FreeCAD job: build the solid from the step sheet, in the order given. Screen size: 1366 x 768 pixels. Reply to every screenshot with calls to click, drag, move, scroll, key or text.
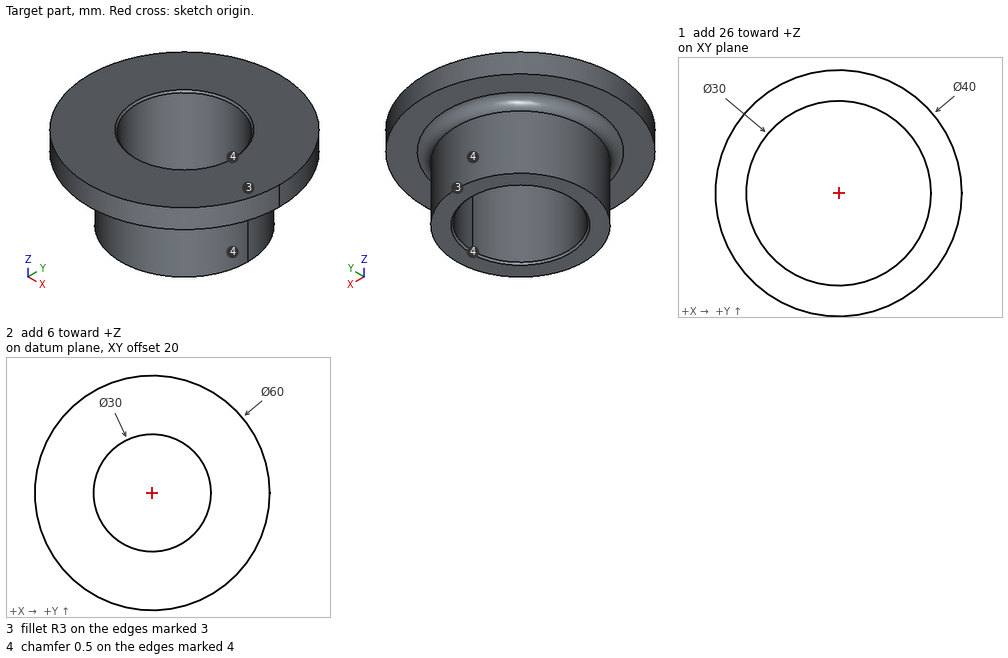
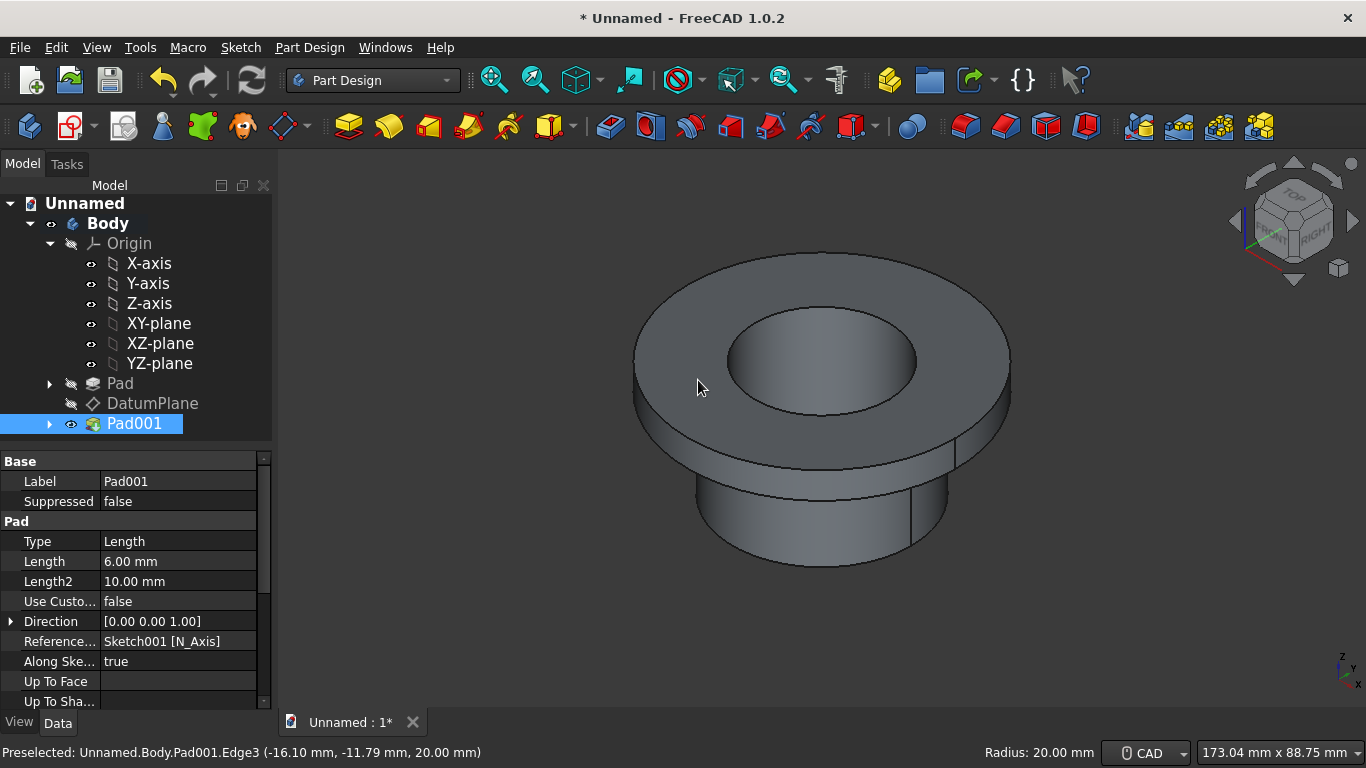
click(966, 126)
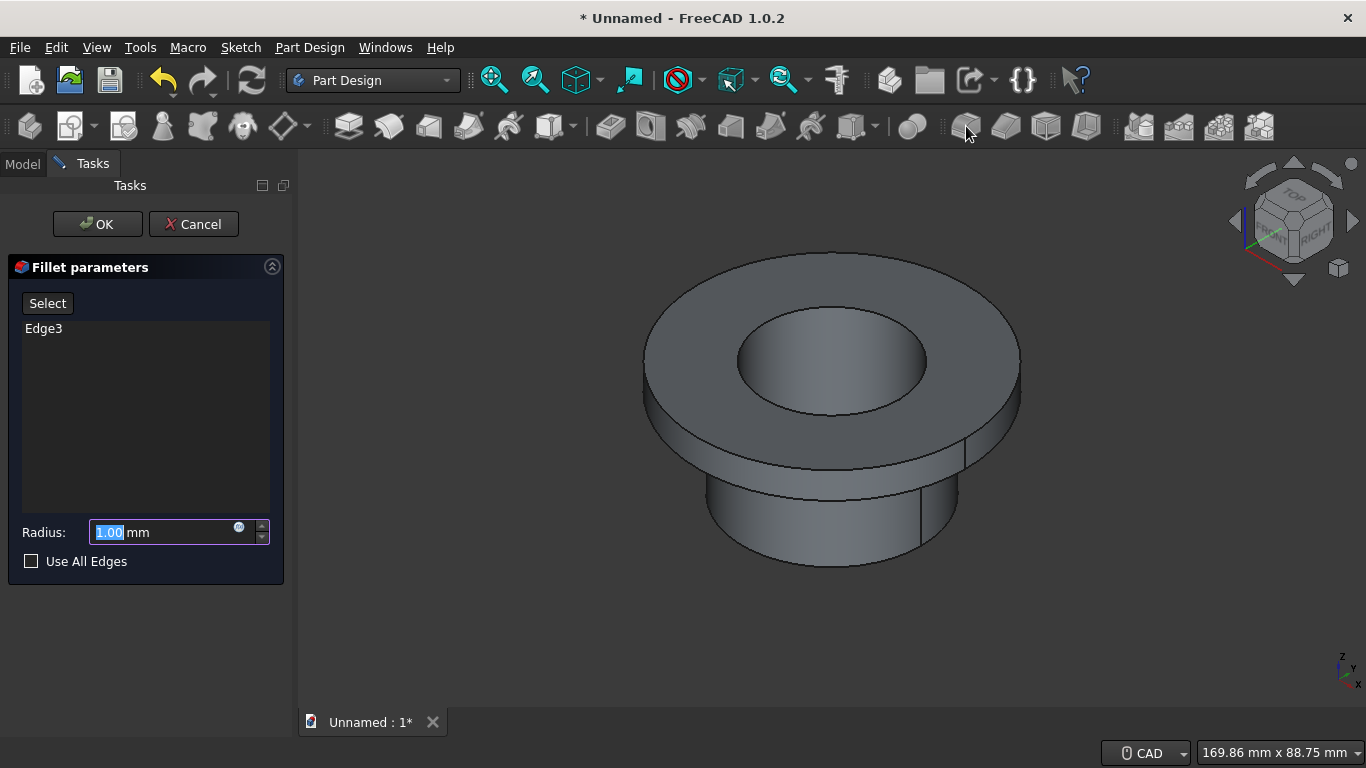
text(3)
key(Tab)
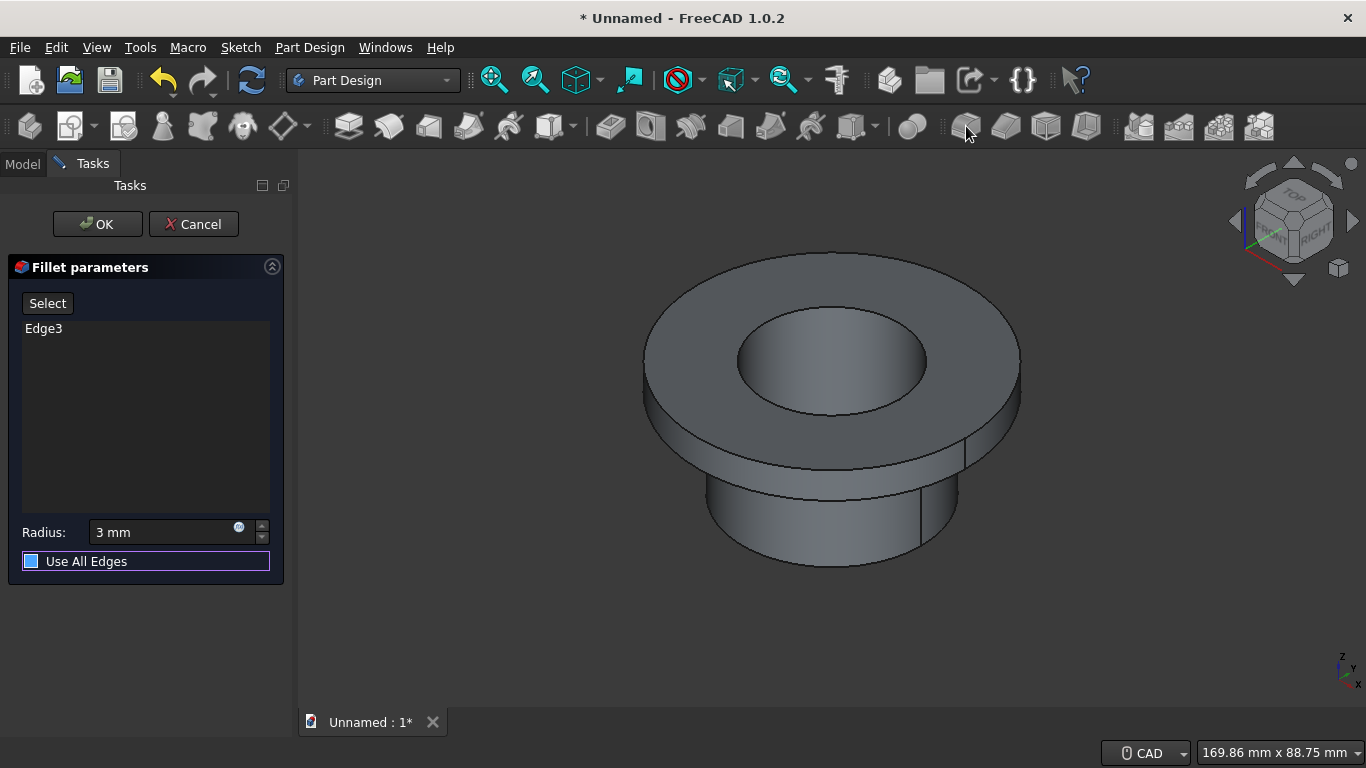
click(98, 224)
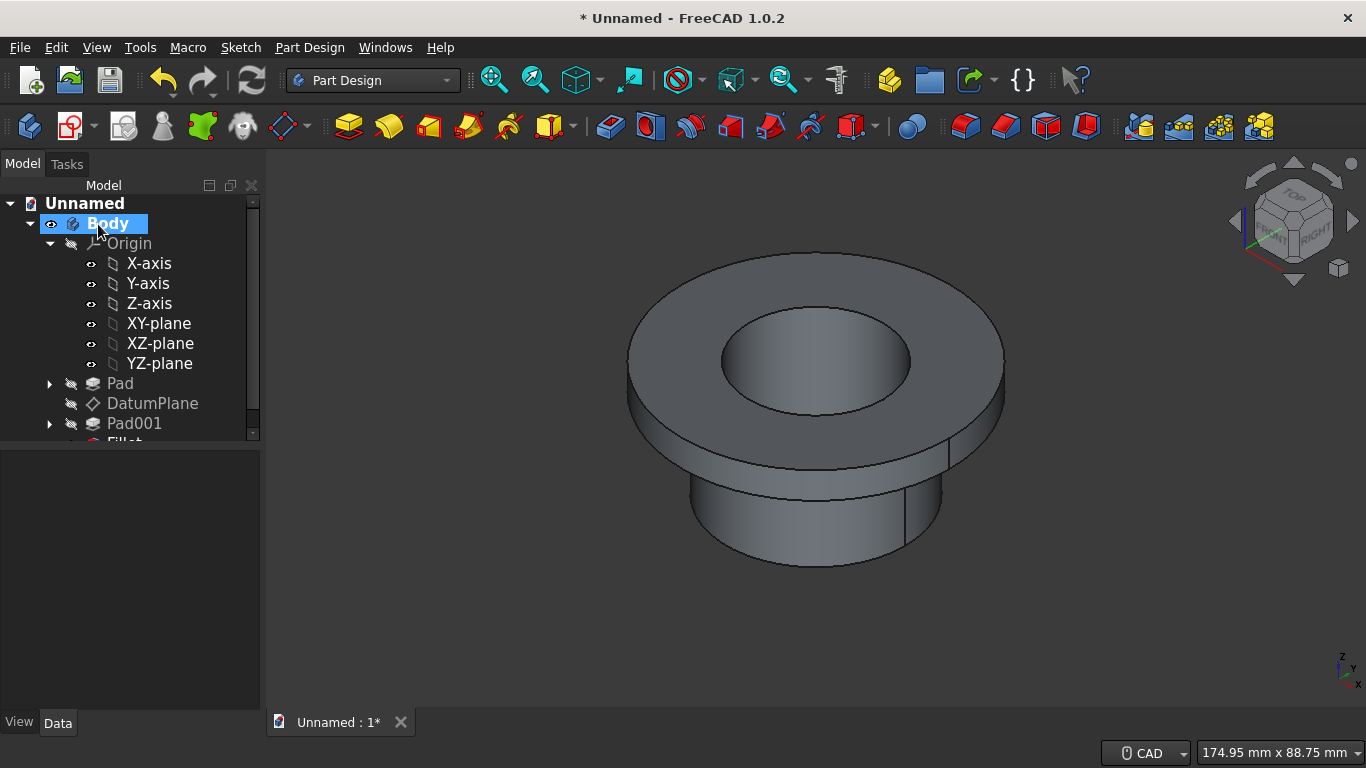
click(749, 322)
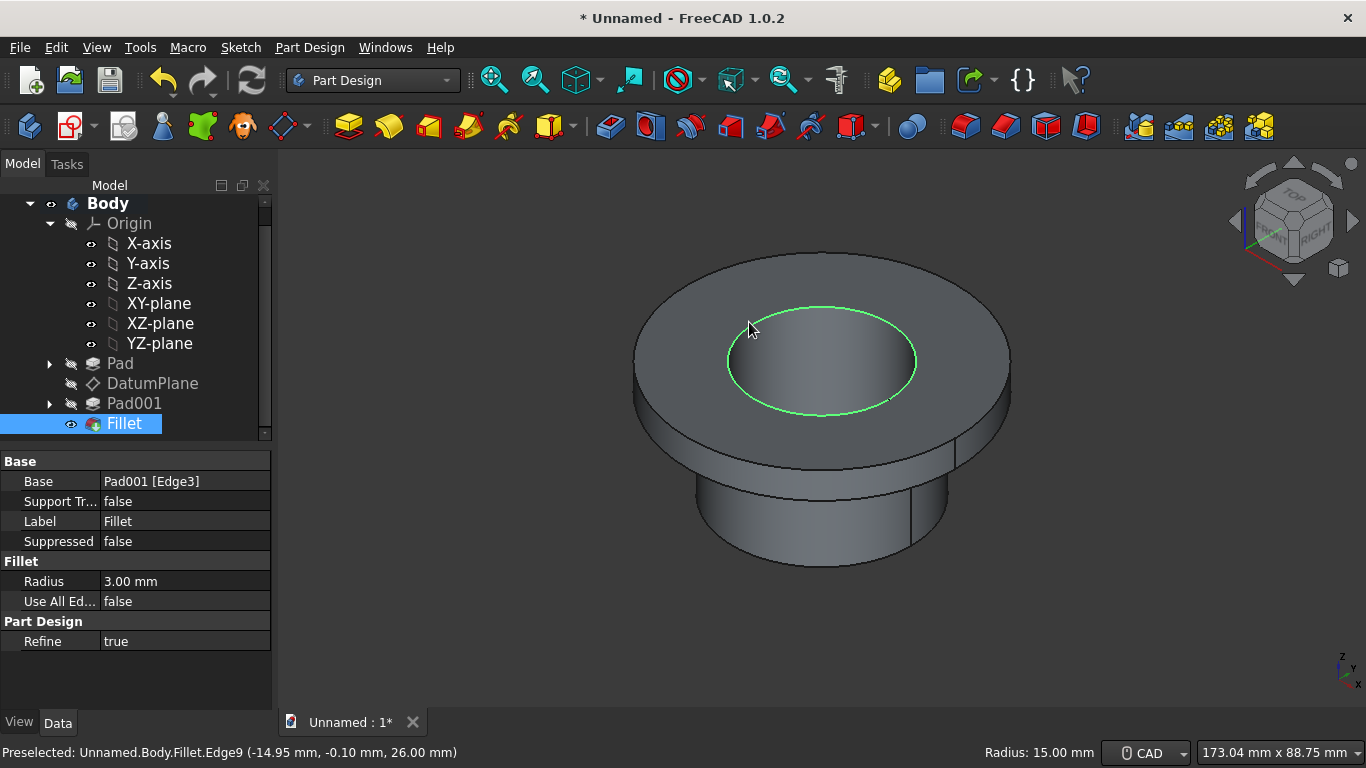
key(2)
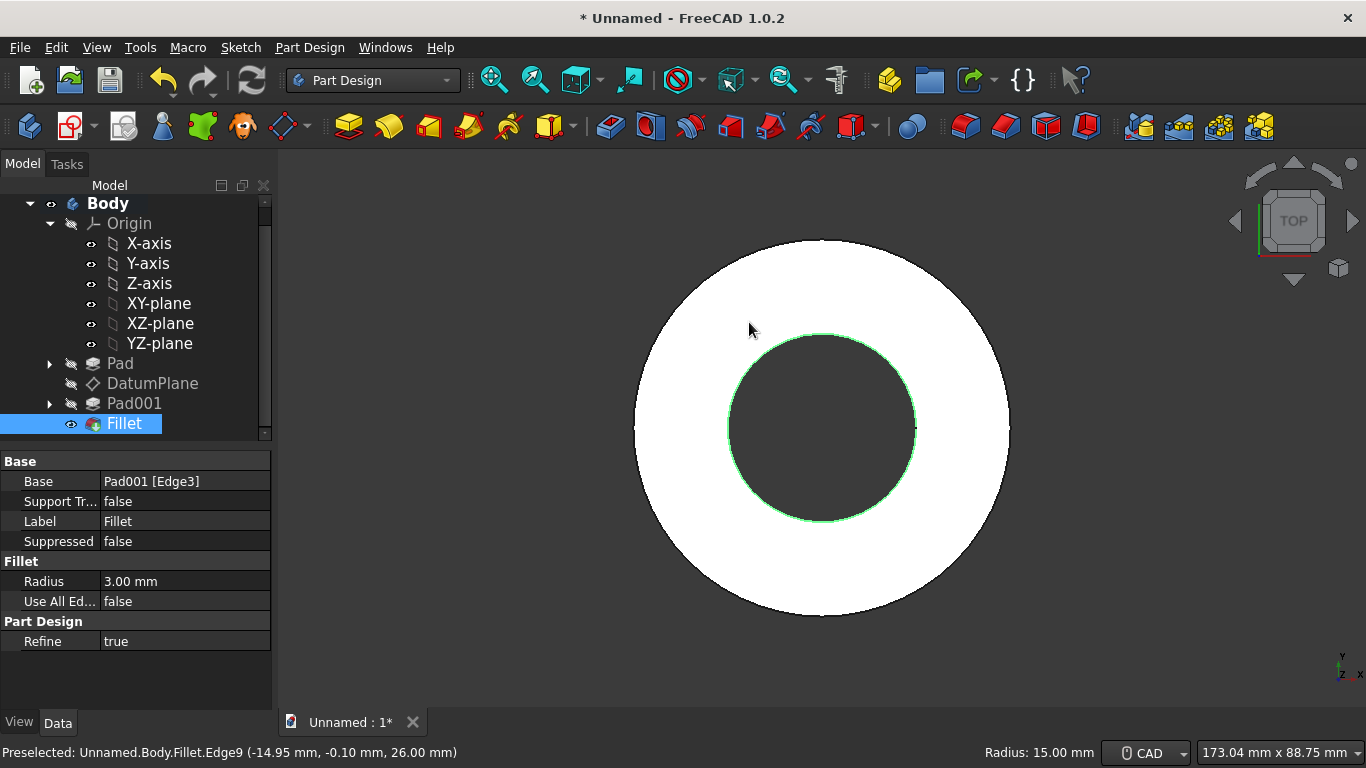
key(0)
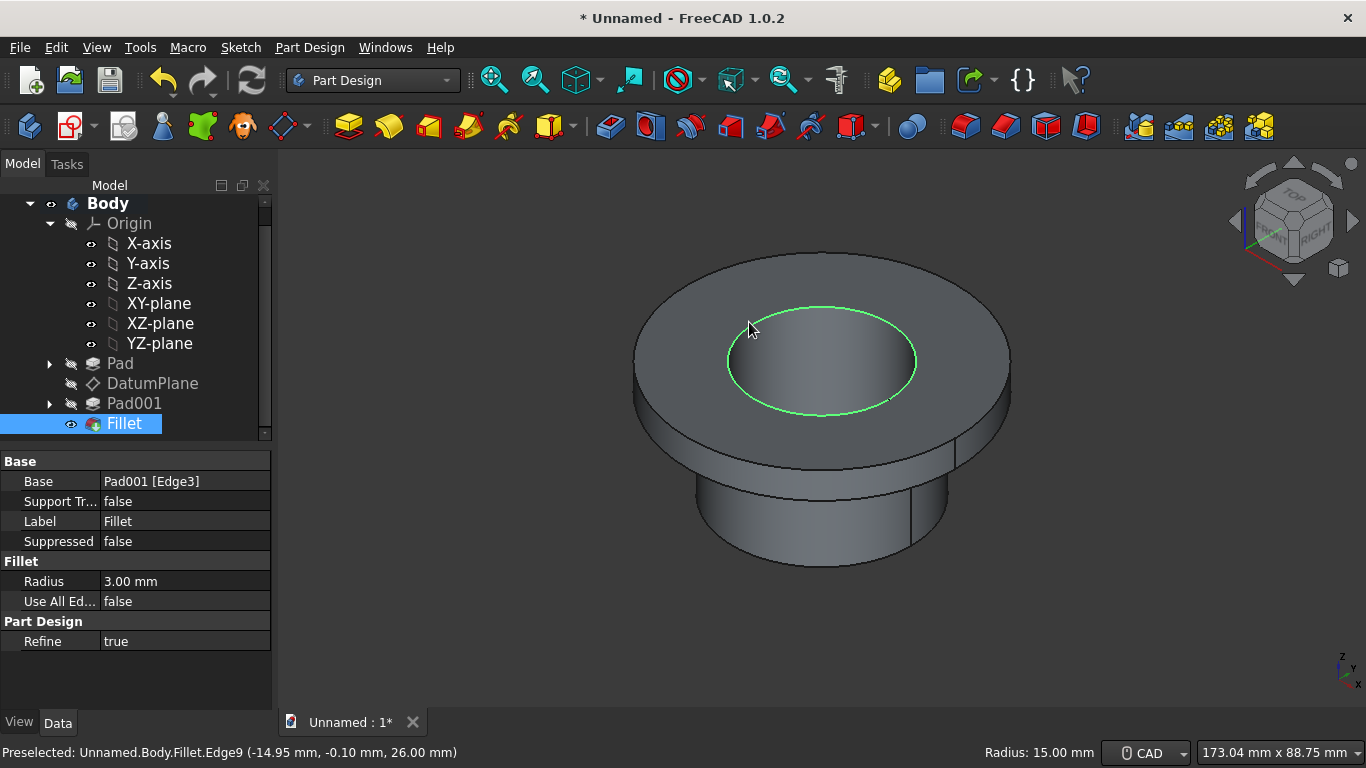
key(1)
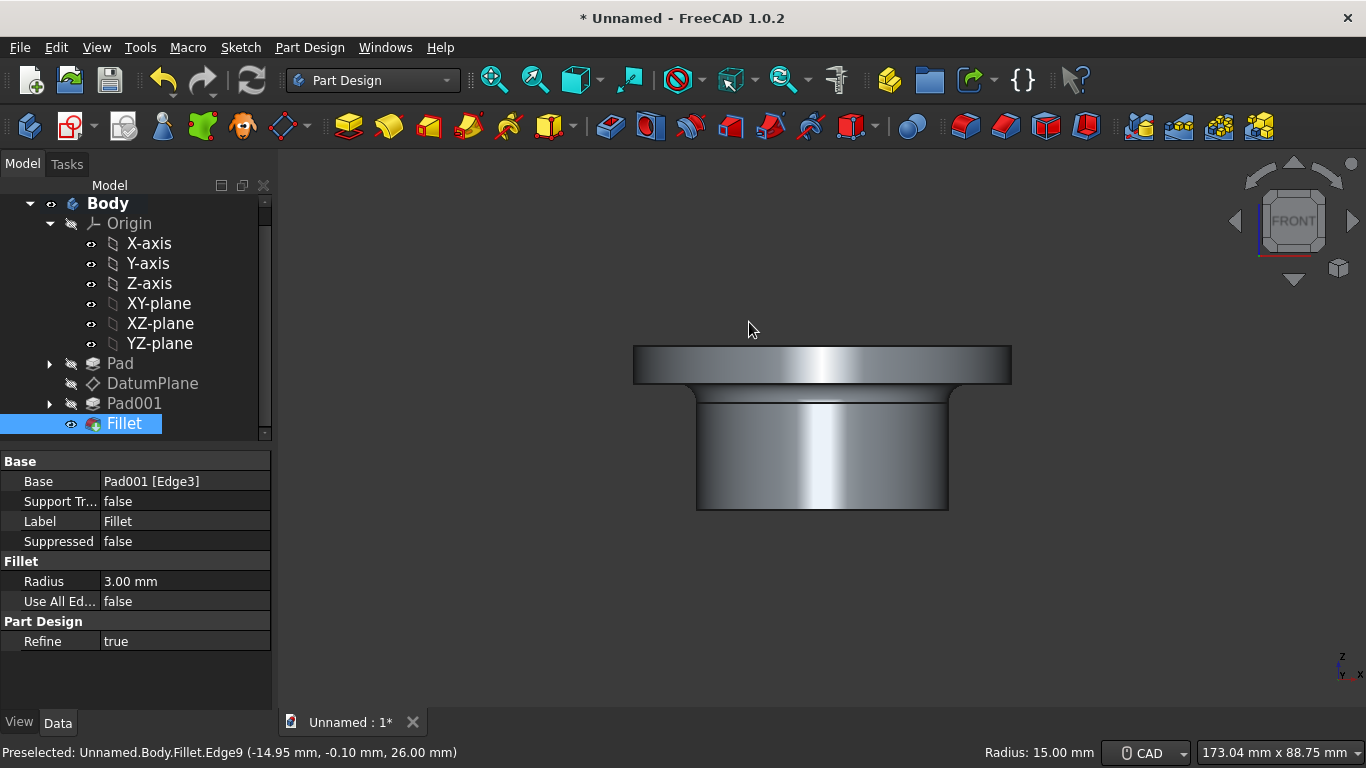
click(496, 80)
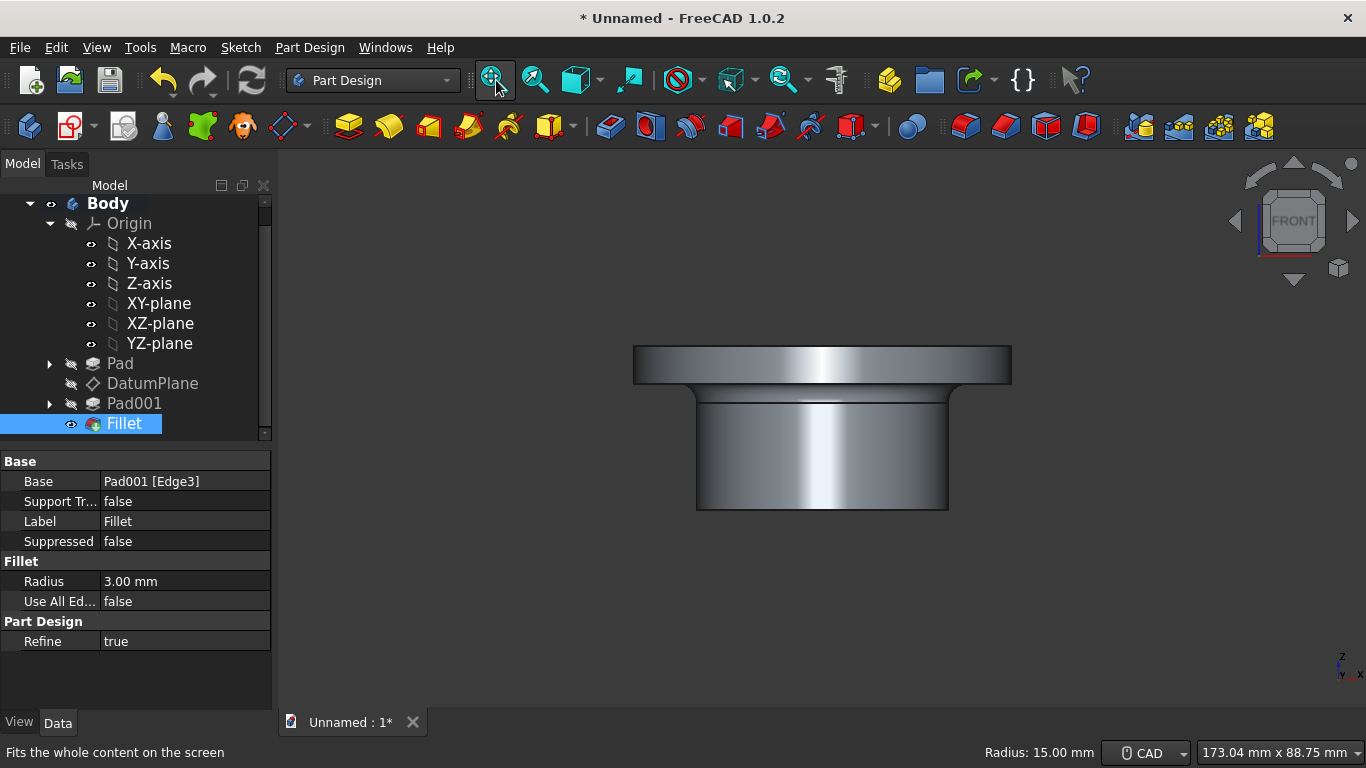
key(3)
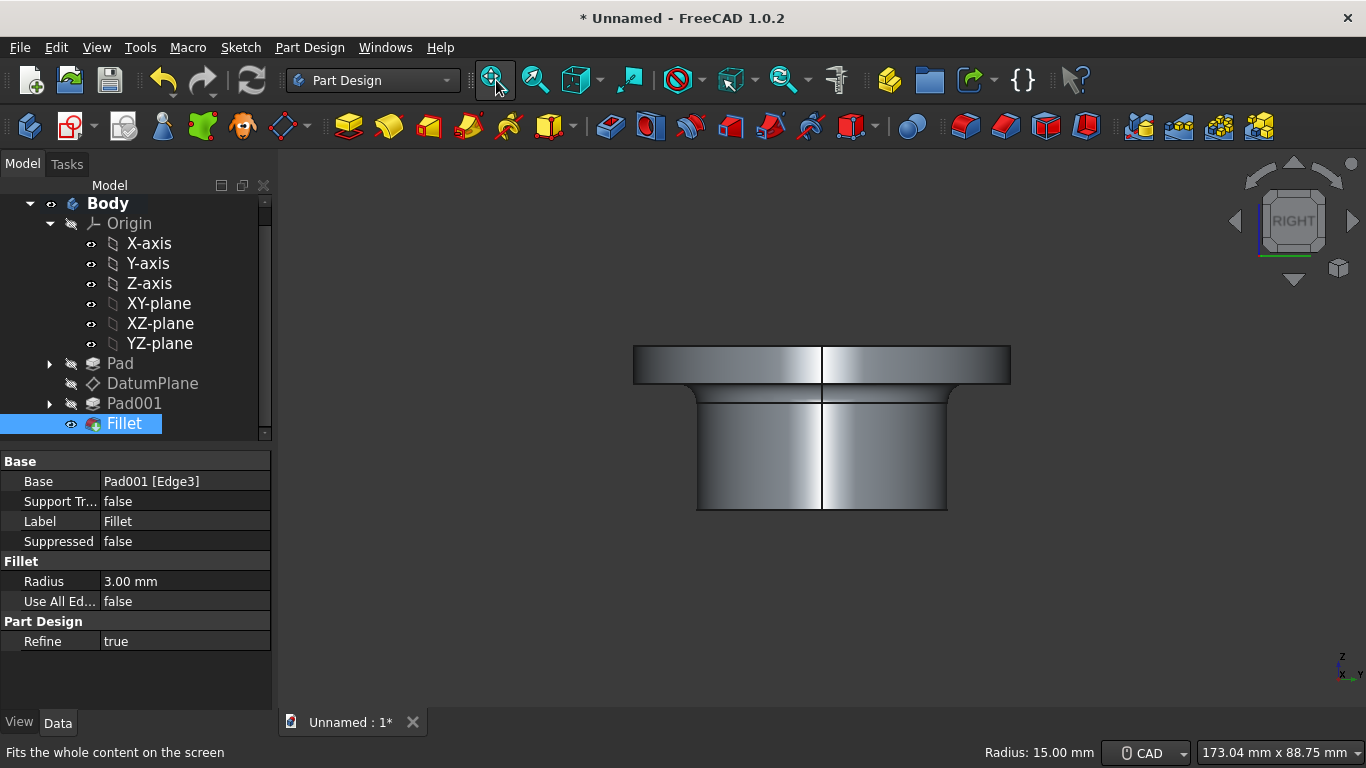
click(496, 80)